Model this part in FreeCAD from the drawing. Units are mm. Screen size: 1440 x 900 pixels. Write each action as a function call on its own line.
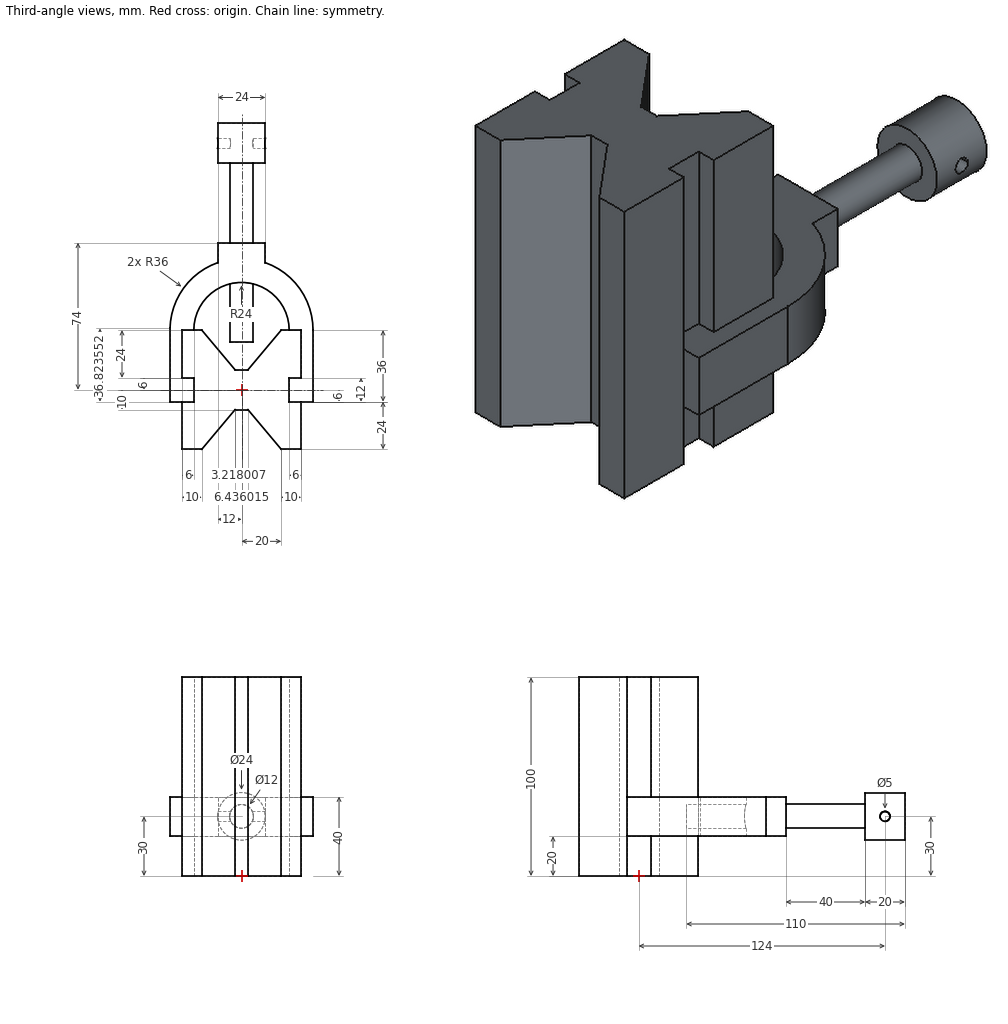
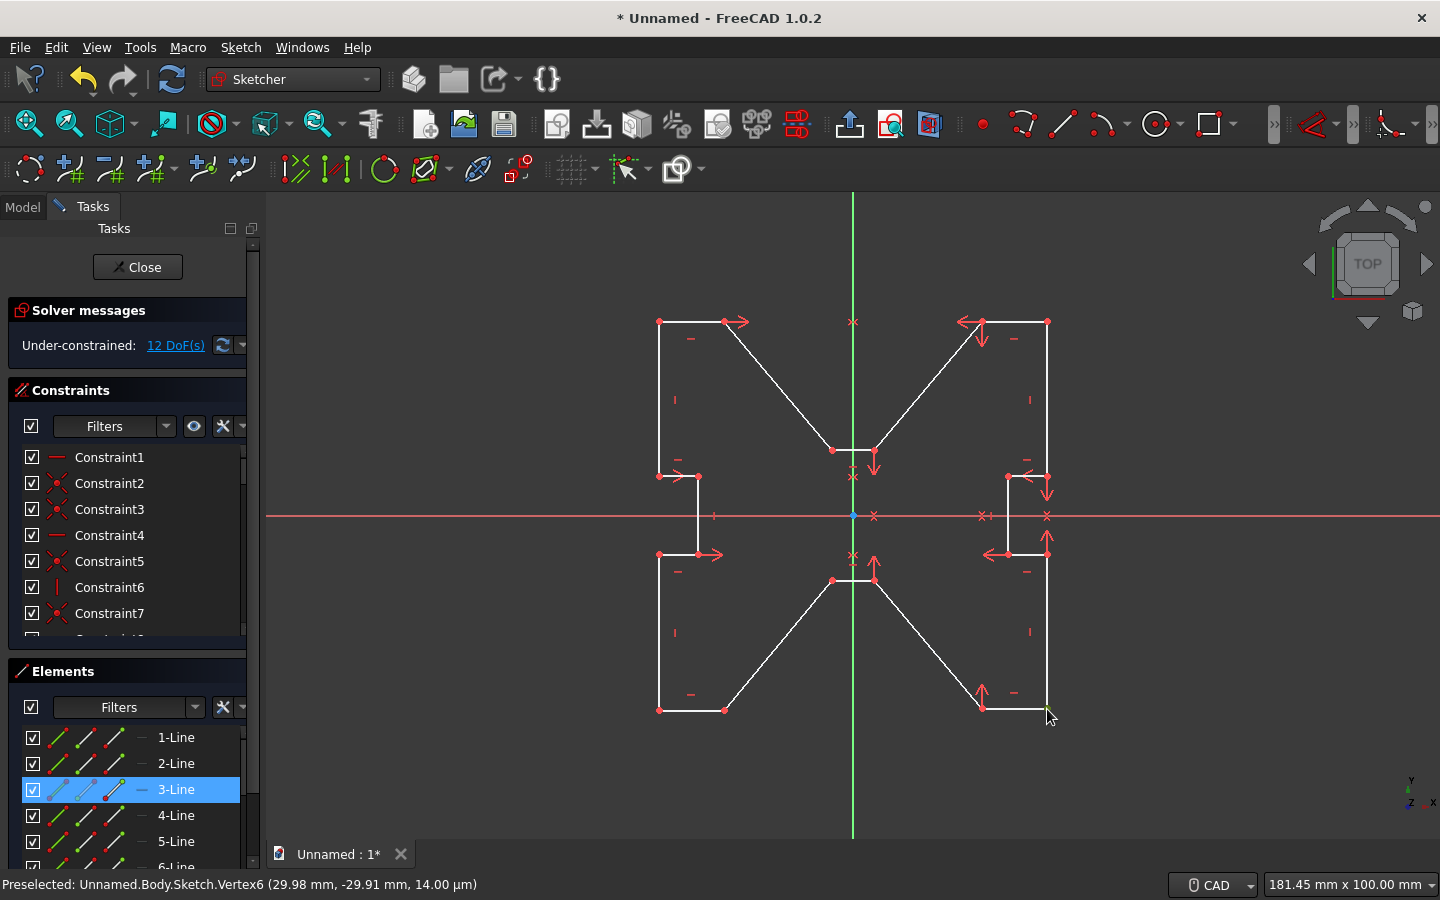
click(659, 711)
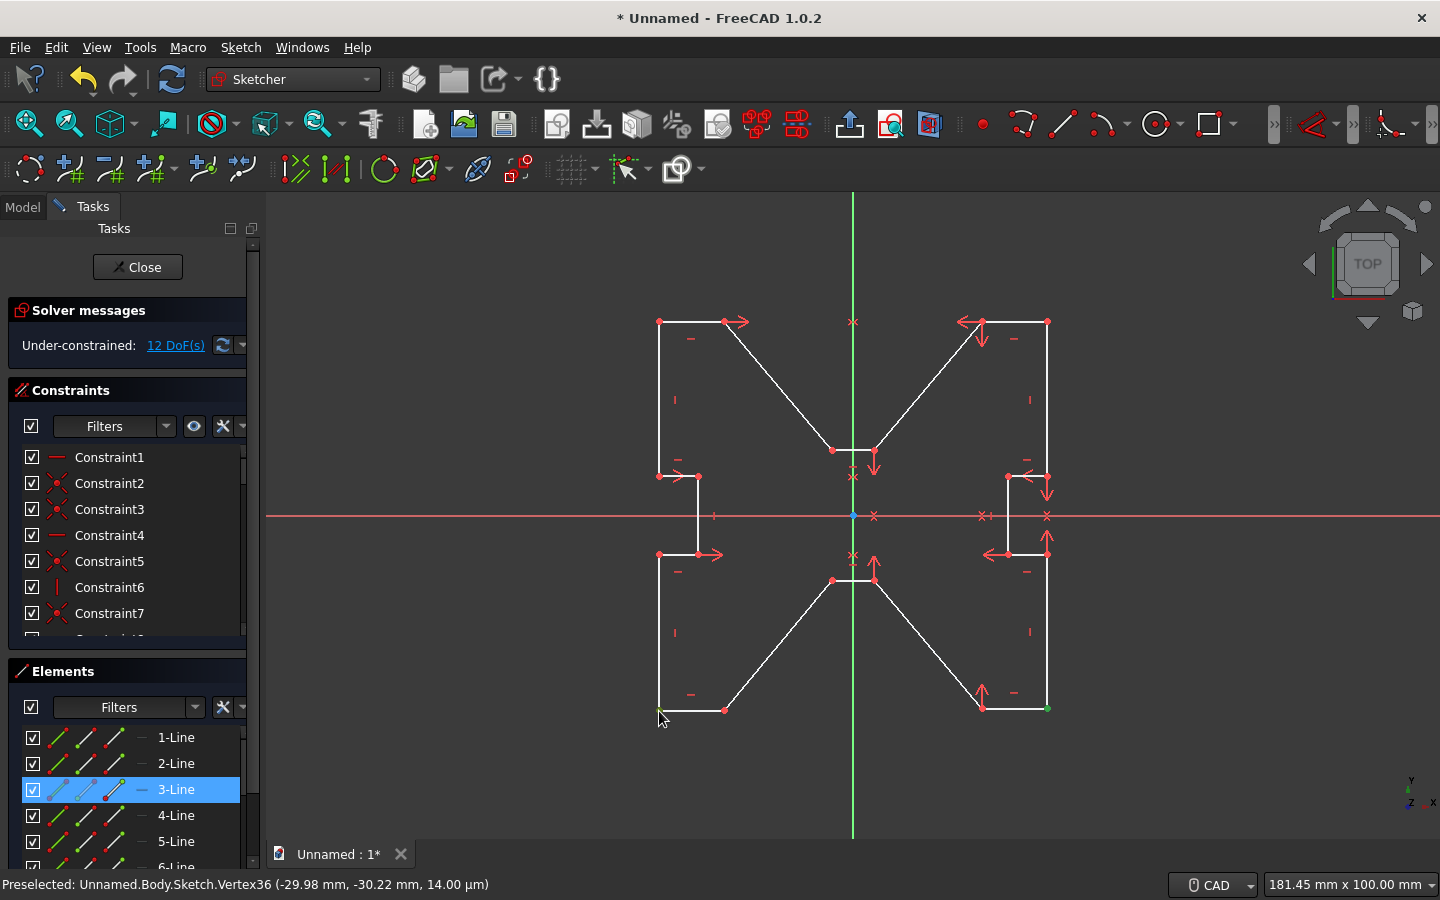
click(853, 769)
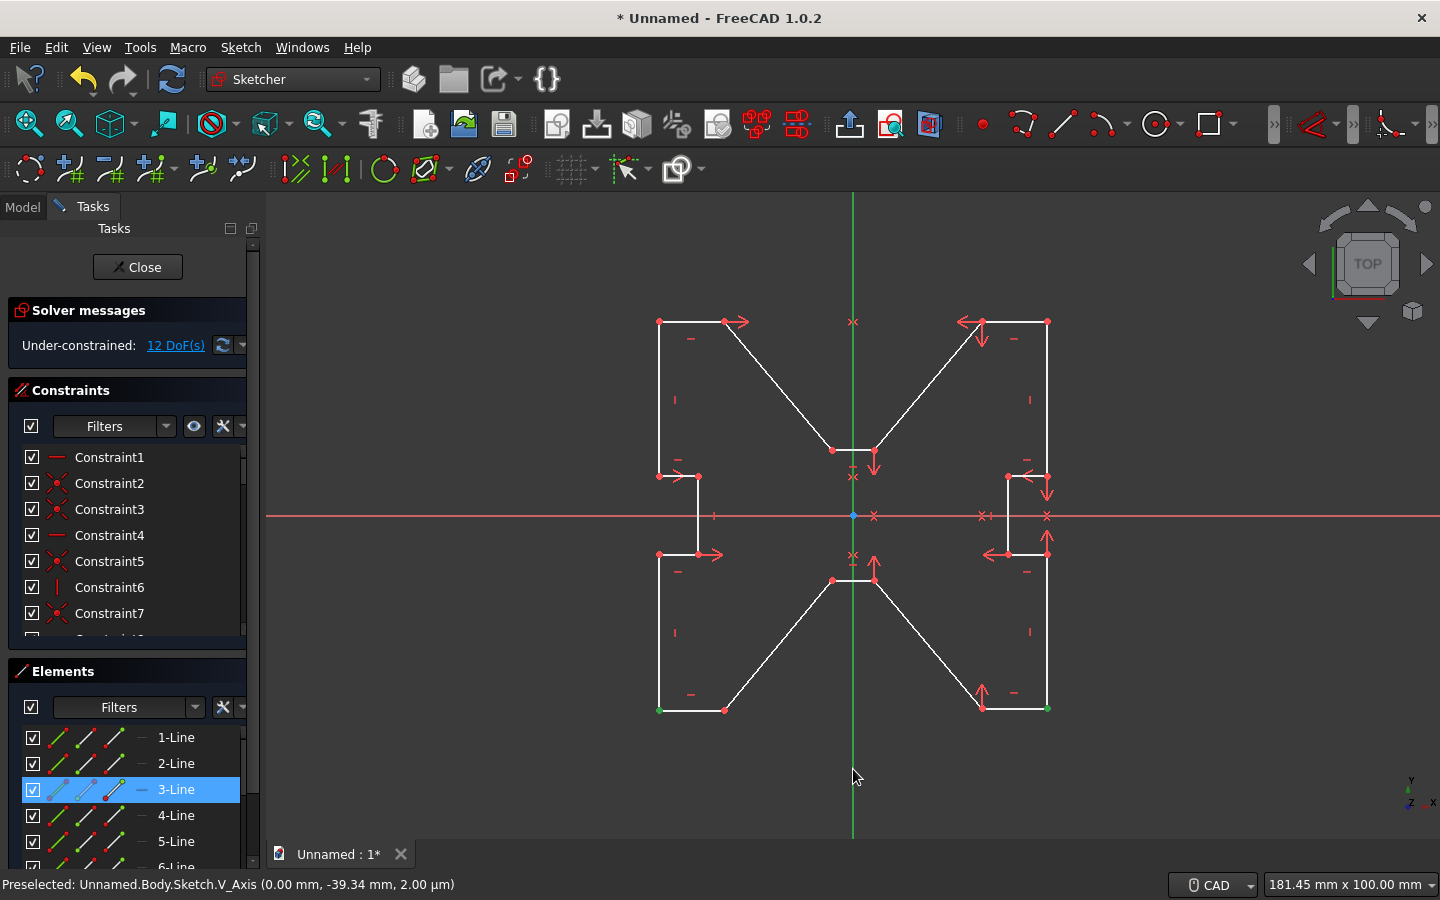
key(s)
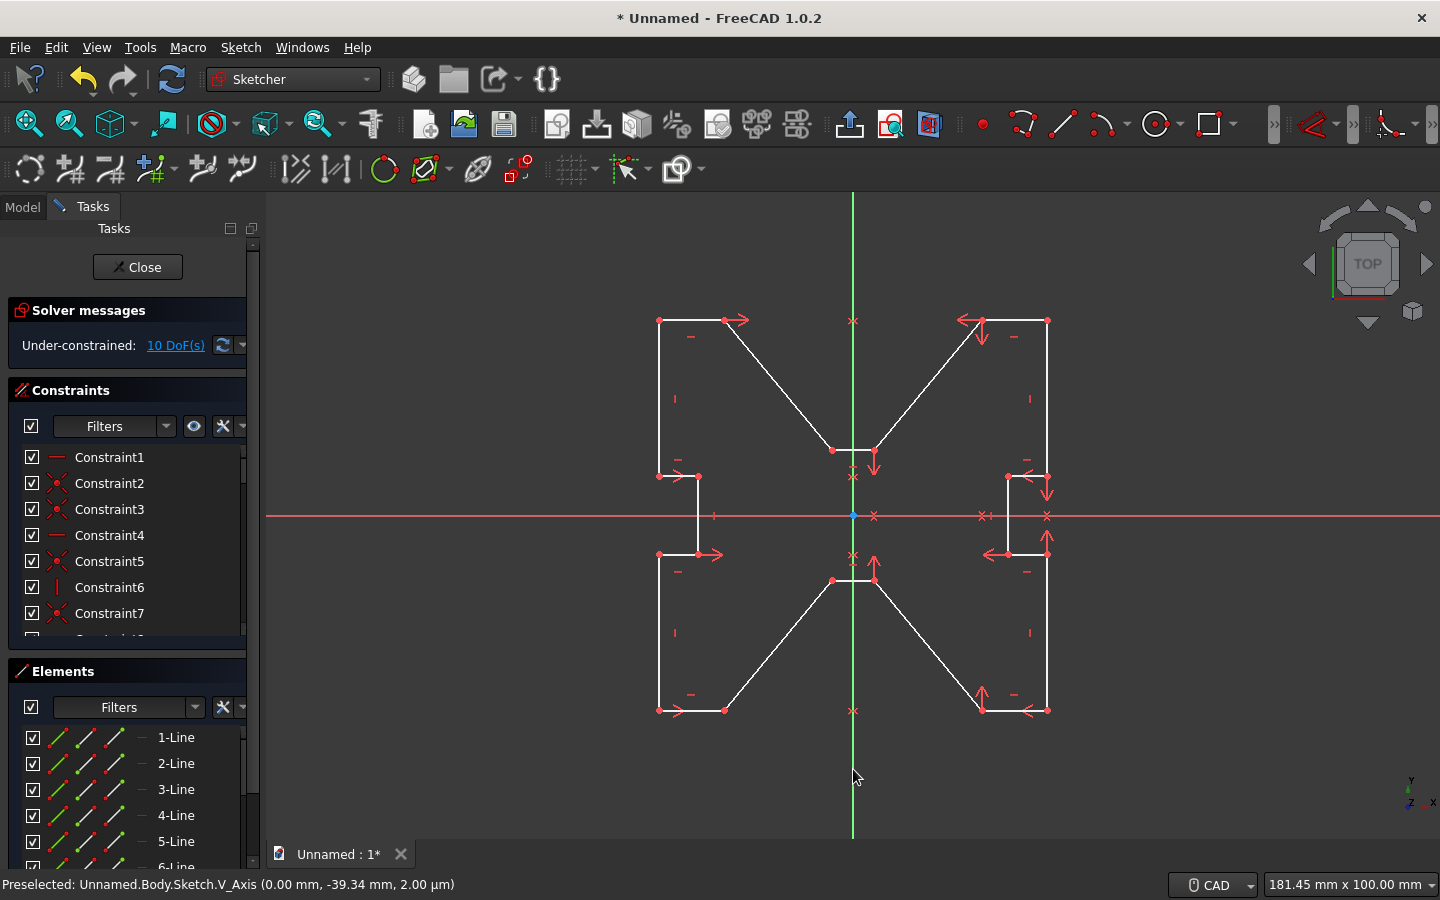
key(d)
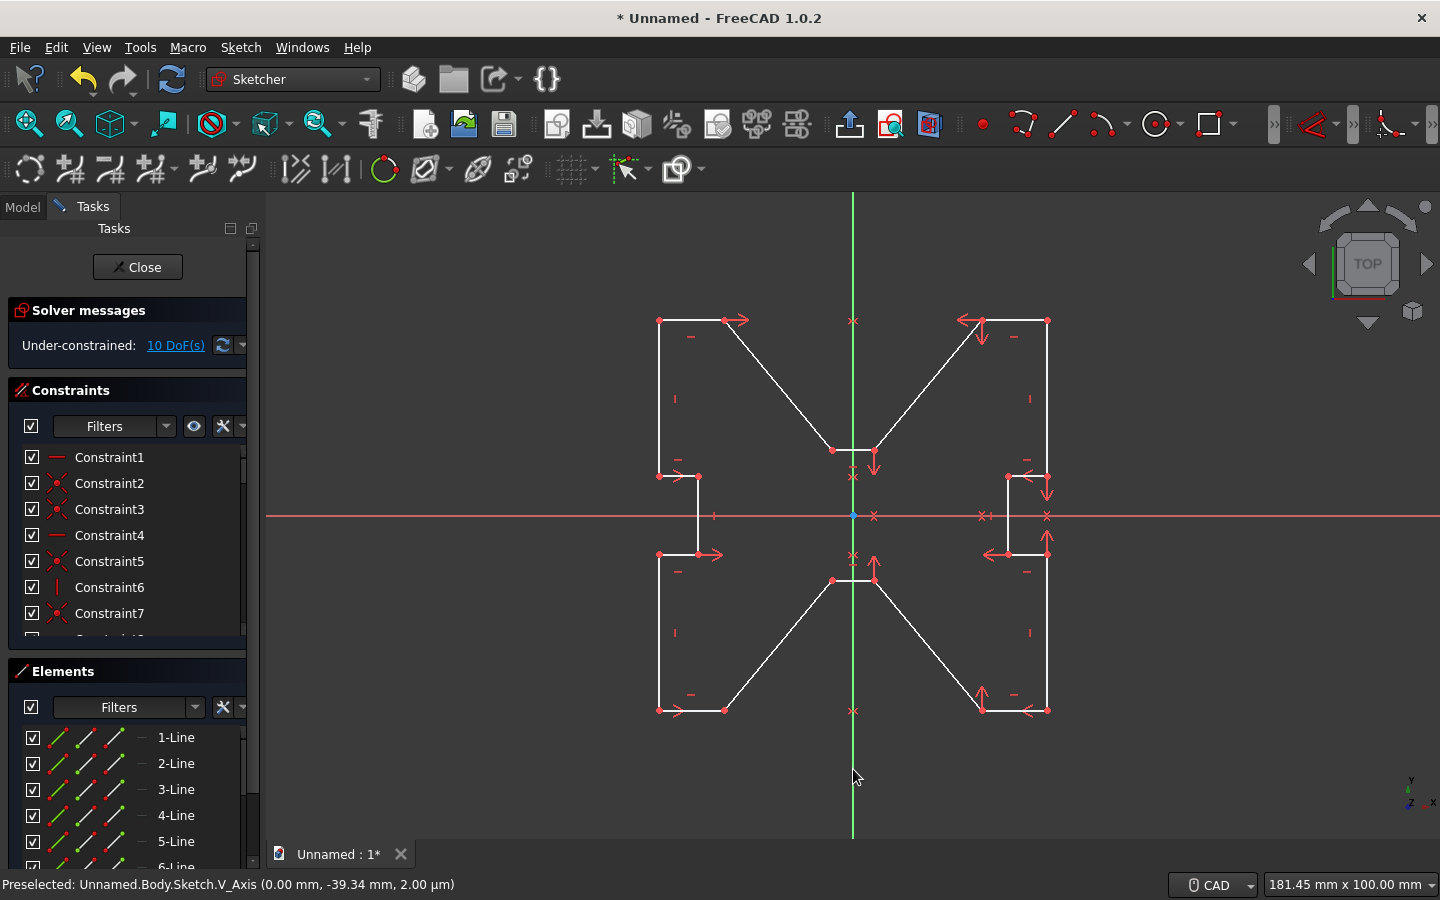
click(1035, 555)
click(1028, 589)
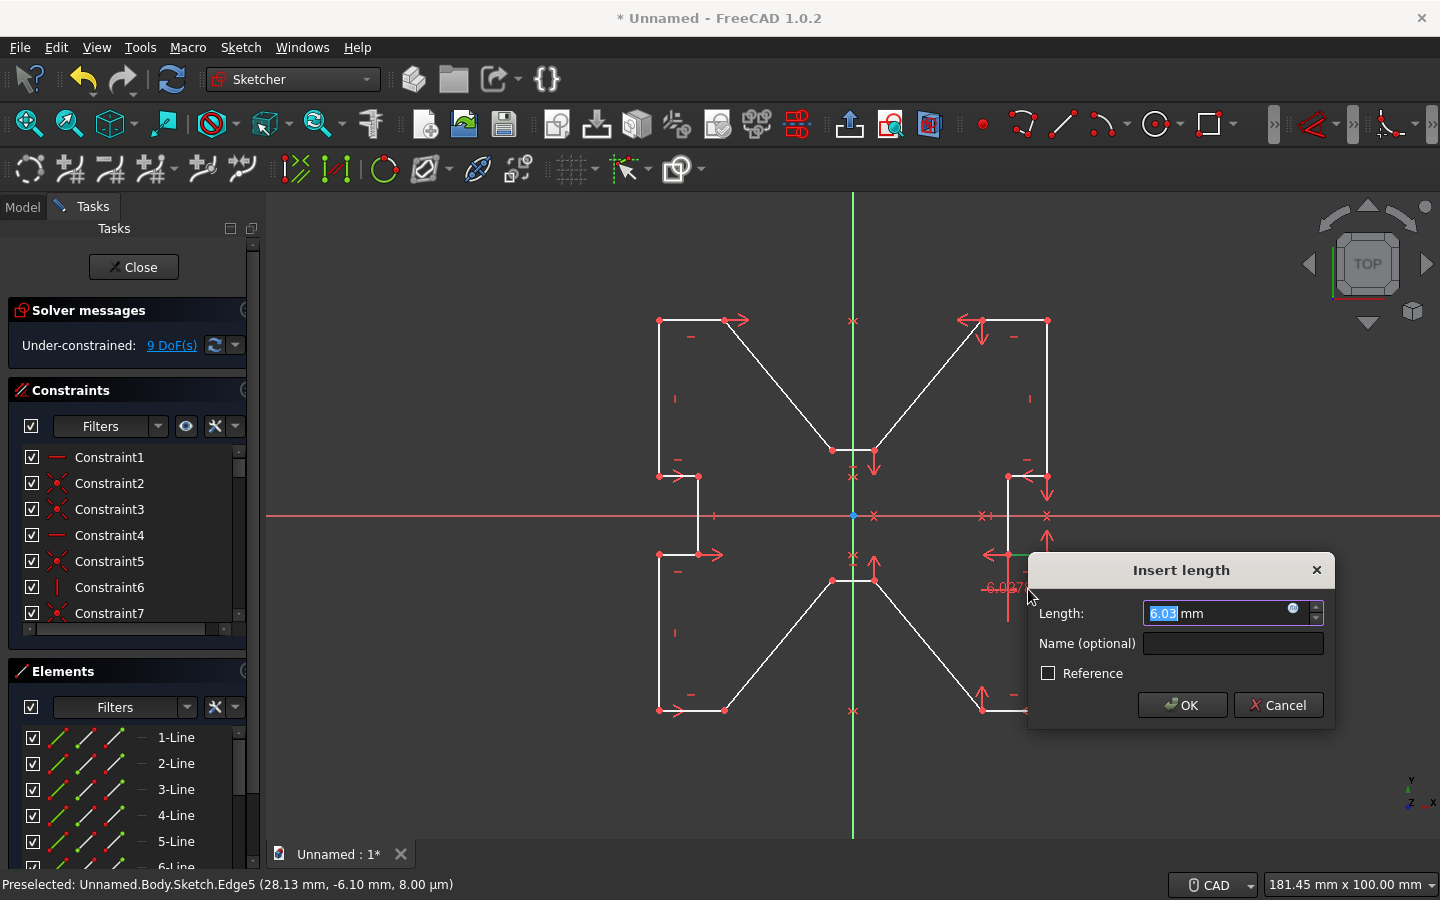
text(6)
key(Return)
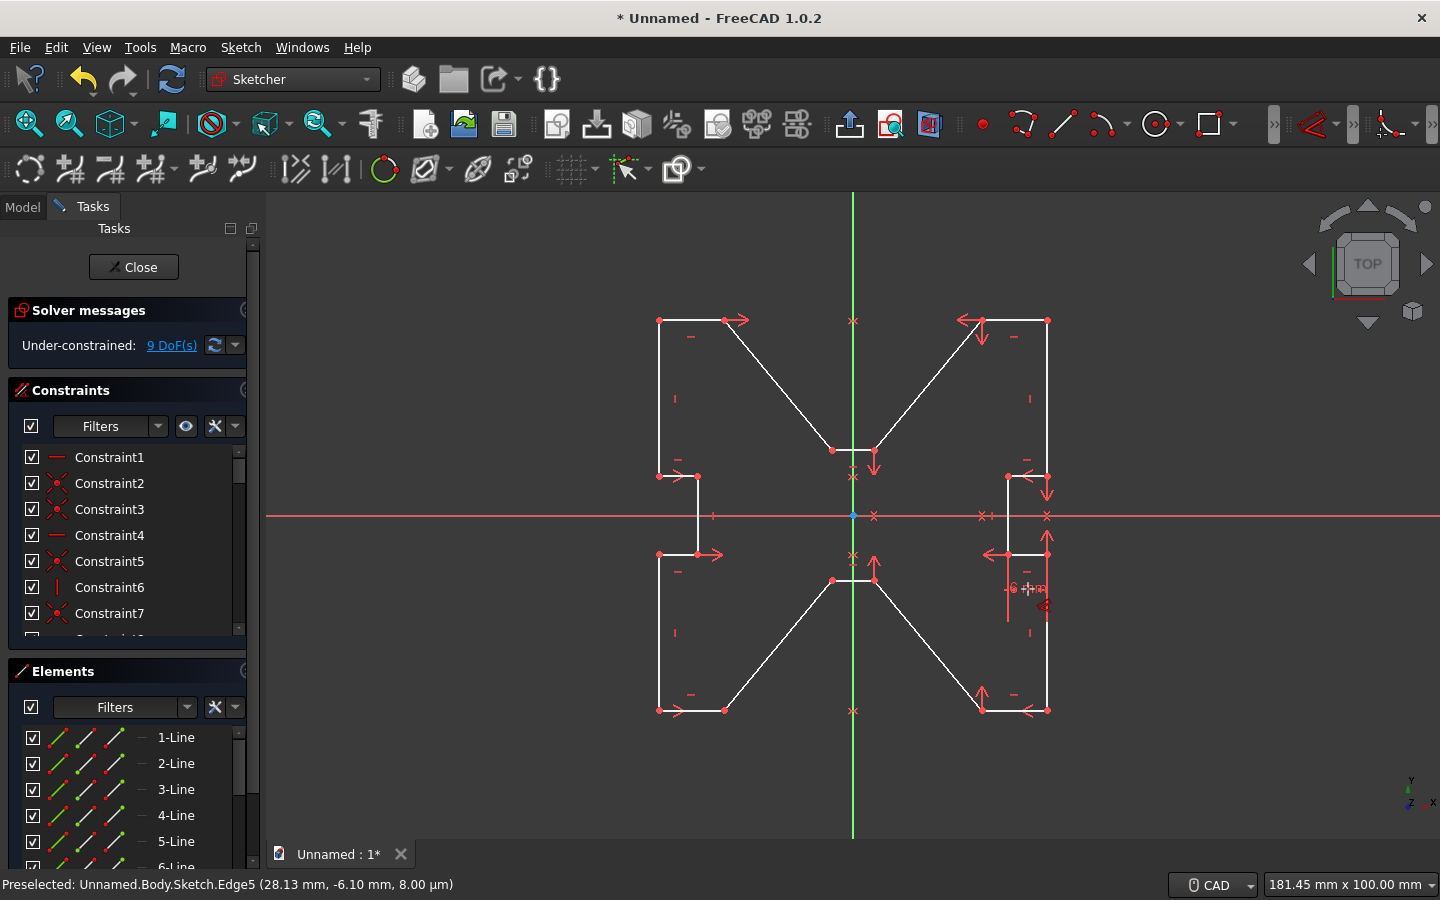
click(1002, 711)
click(1015, 745)